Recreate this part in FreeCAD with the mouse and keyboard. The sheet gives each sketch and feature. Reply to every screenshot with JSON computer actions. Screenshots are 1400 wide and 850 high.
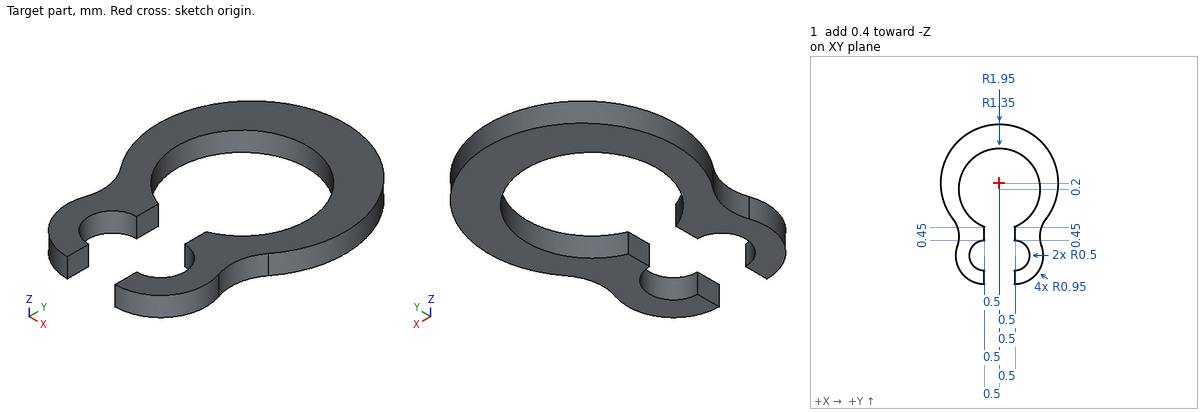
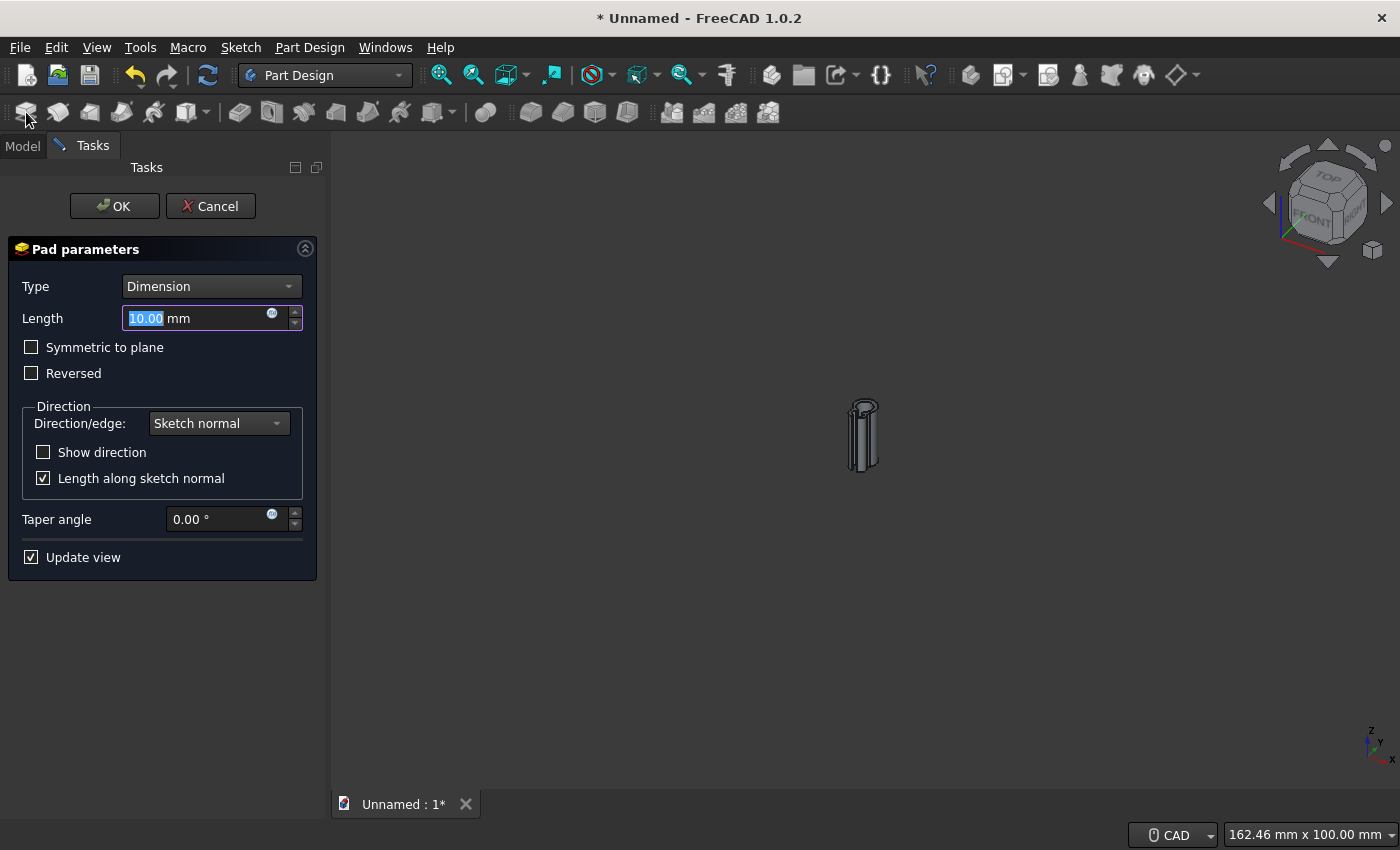
{"action": "type", "text": "0.4"}
{"action": "key", "text": "Tab"}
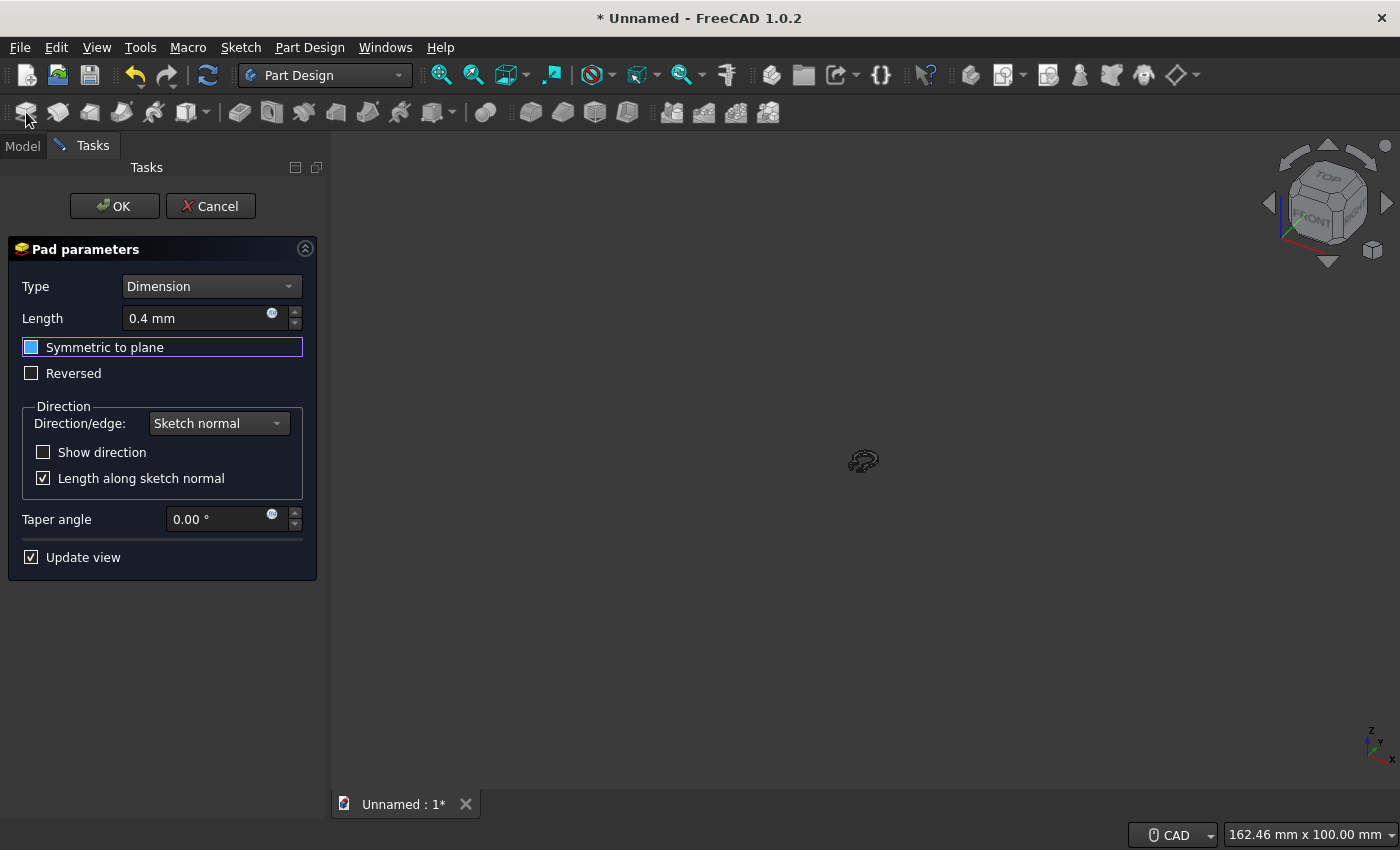
{"action": "left_click", "coordinate": [30, 373]}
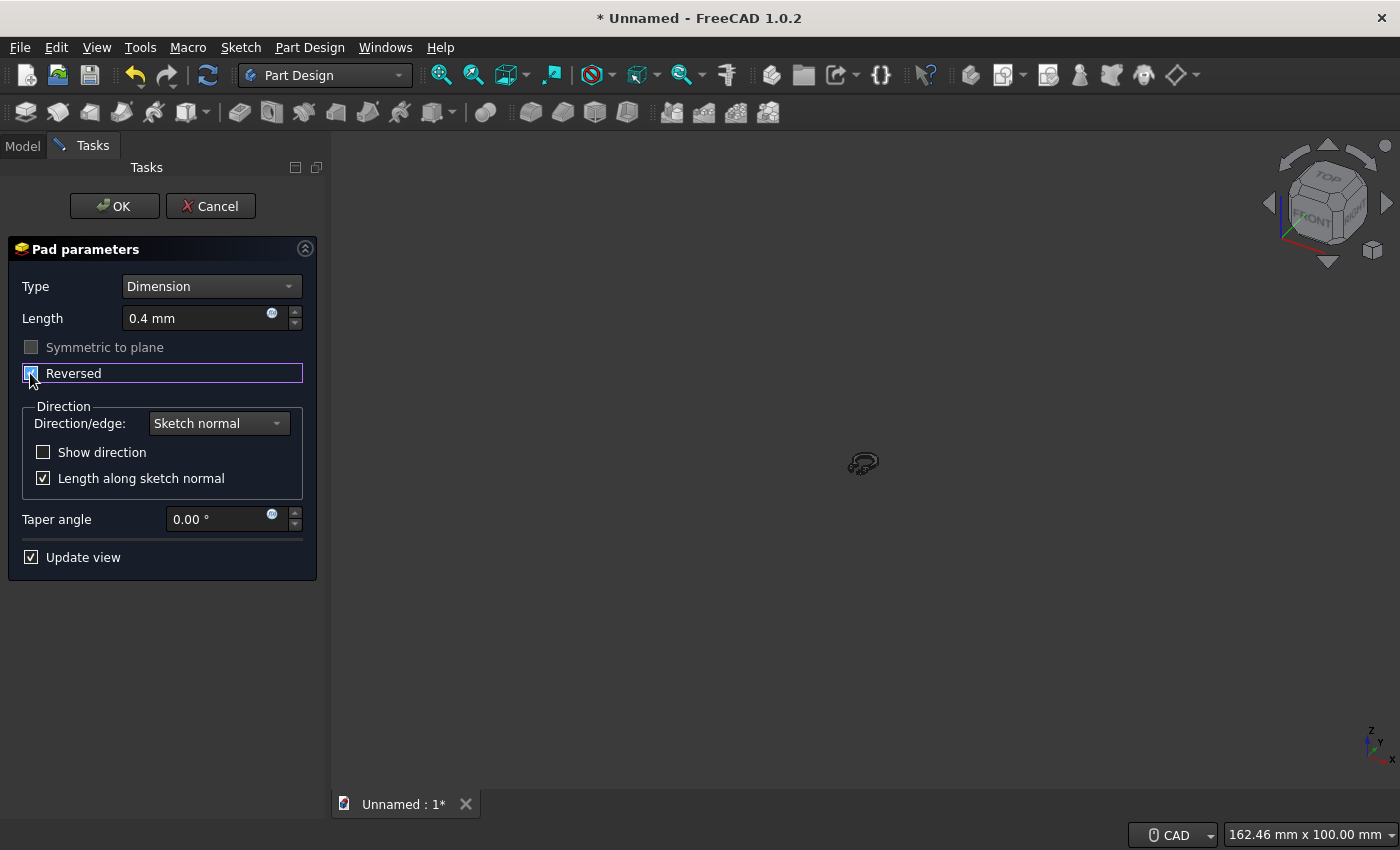
{"action": "left_click", "coordinate": [115, 206]}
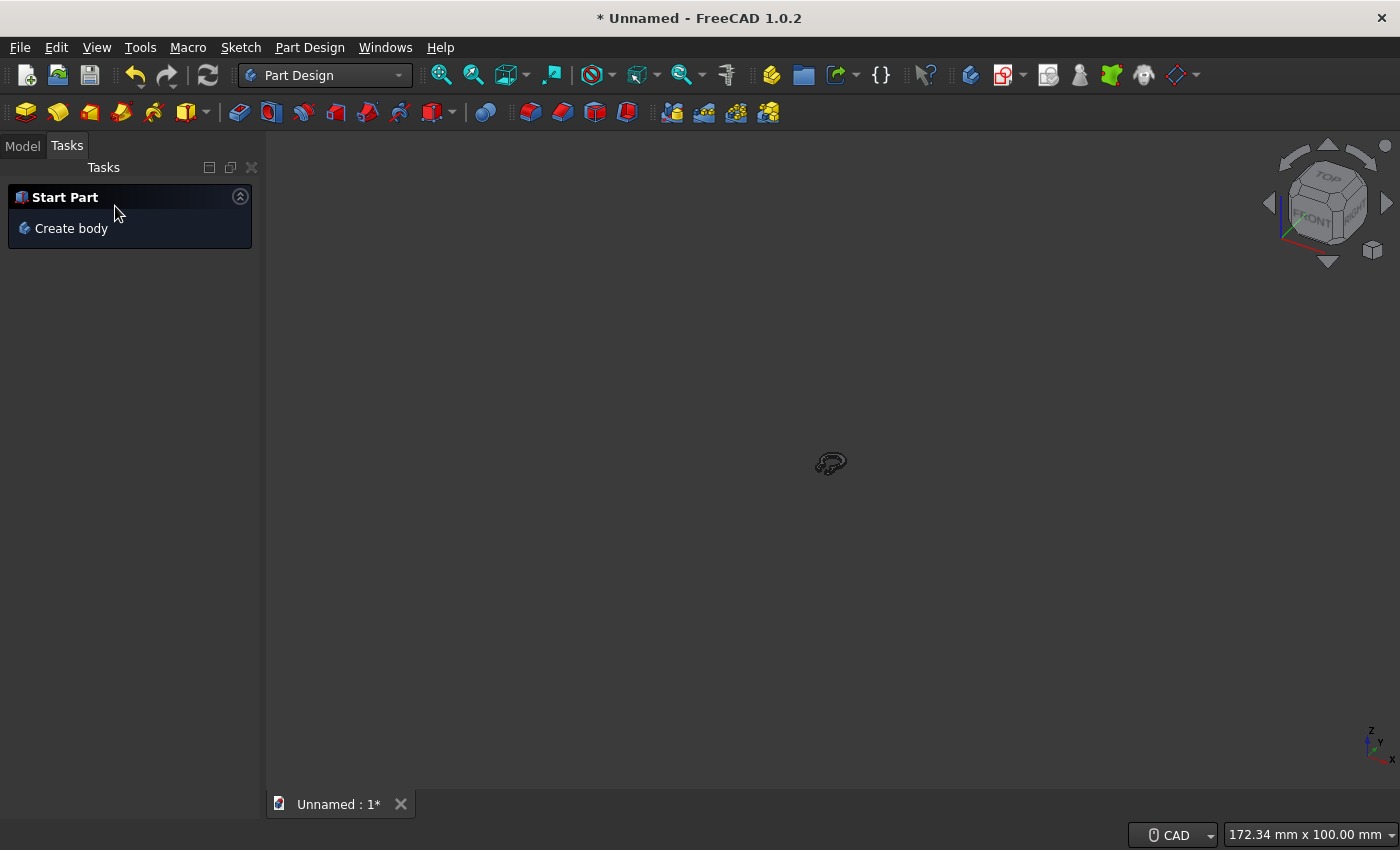
{"action": "key", "text": "0"}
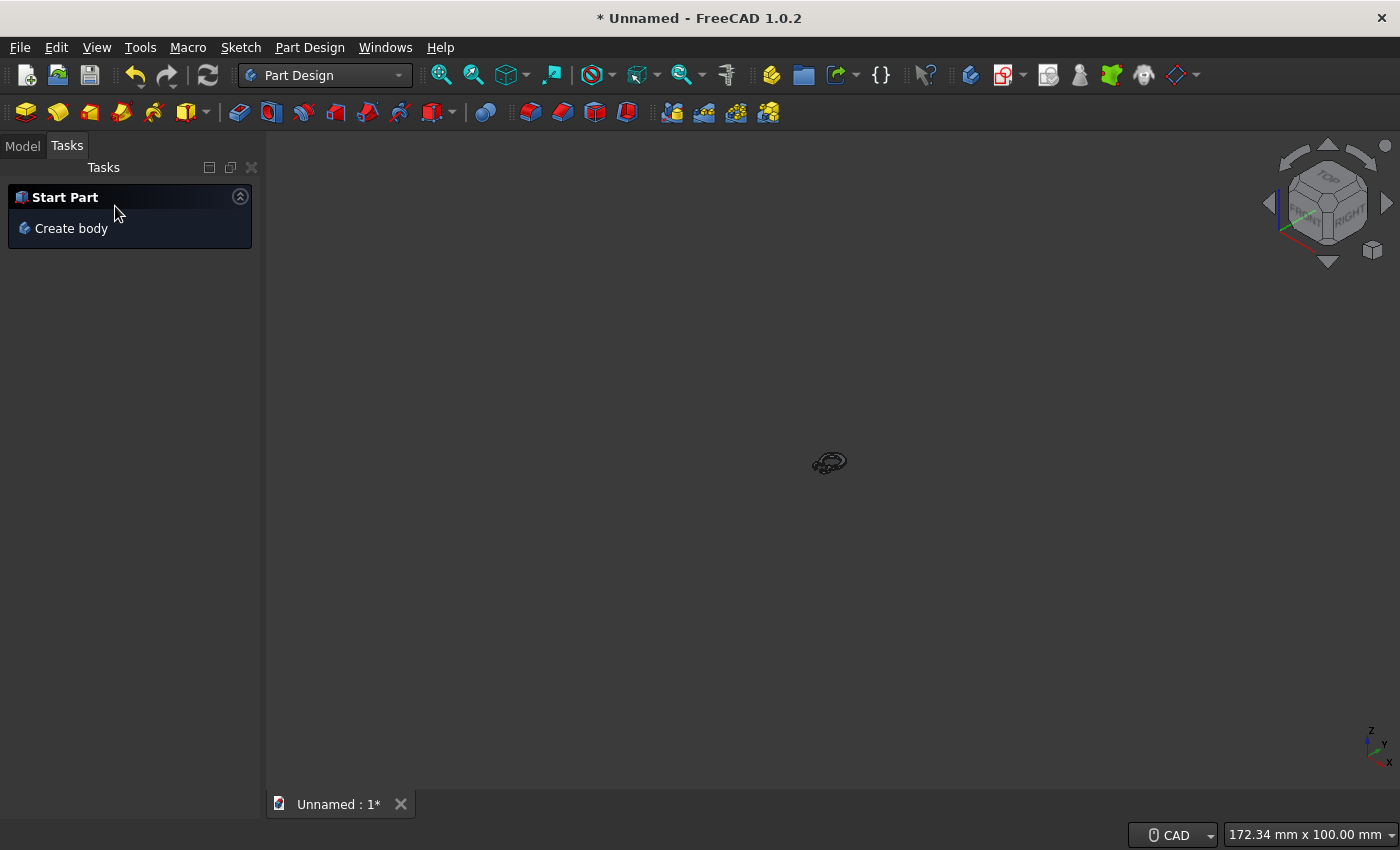
{"action": "key", "text": "v f"}